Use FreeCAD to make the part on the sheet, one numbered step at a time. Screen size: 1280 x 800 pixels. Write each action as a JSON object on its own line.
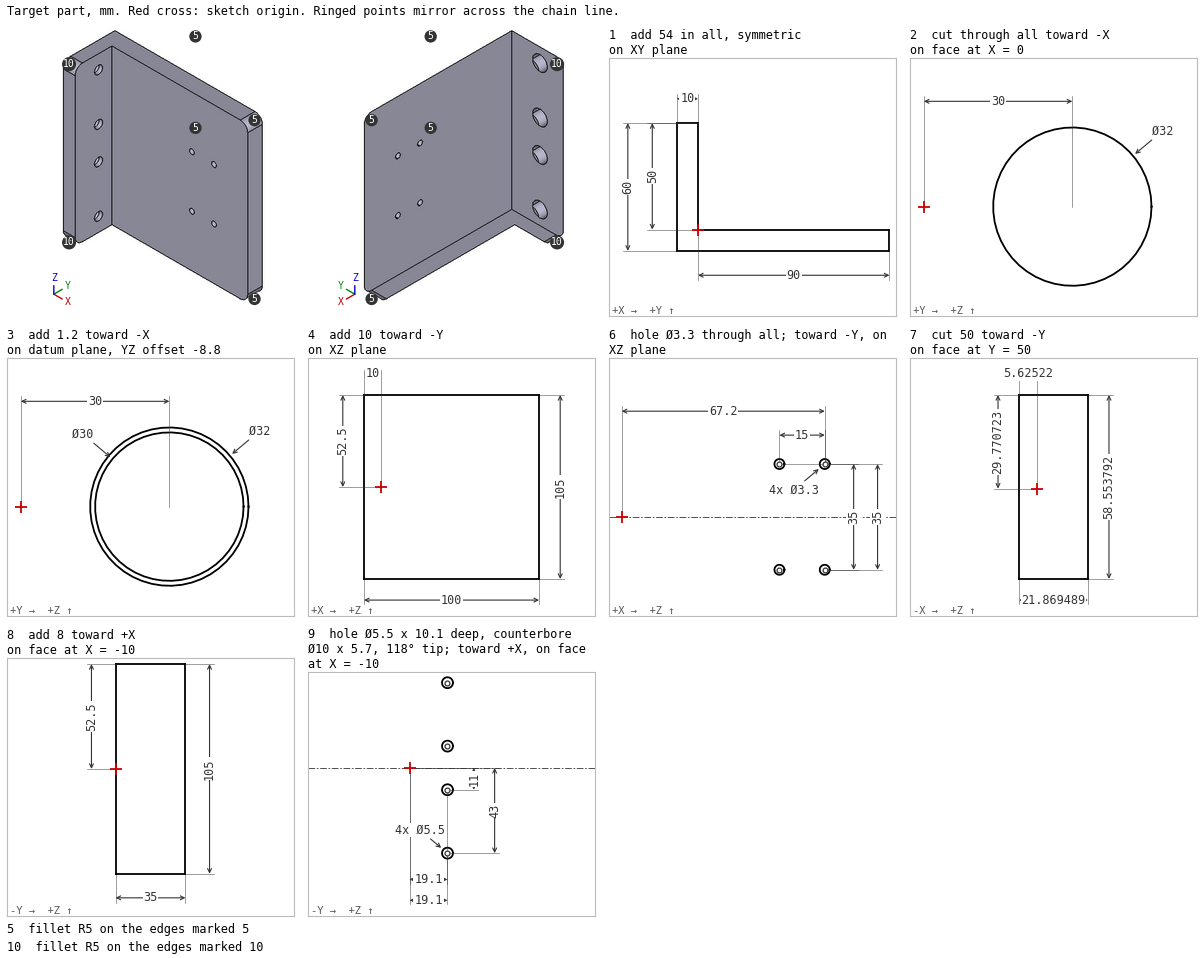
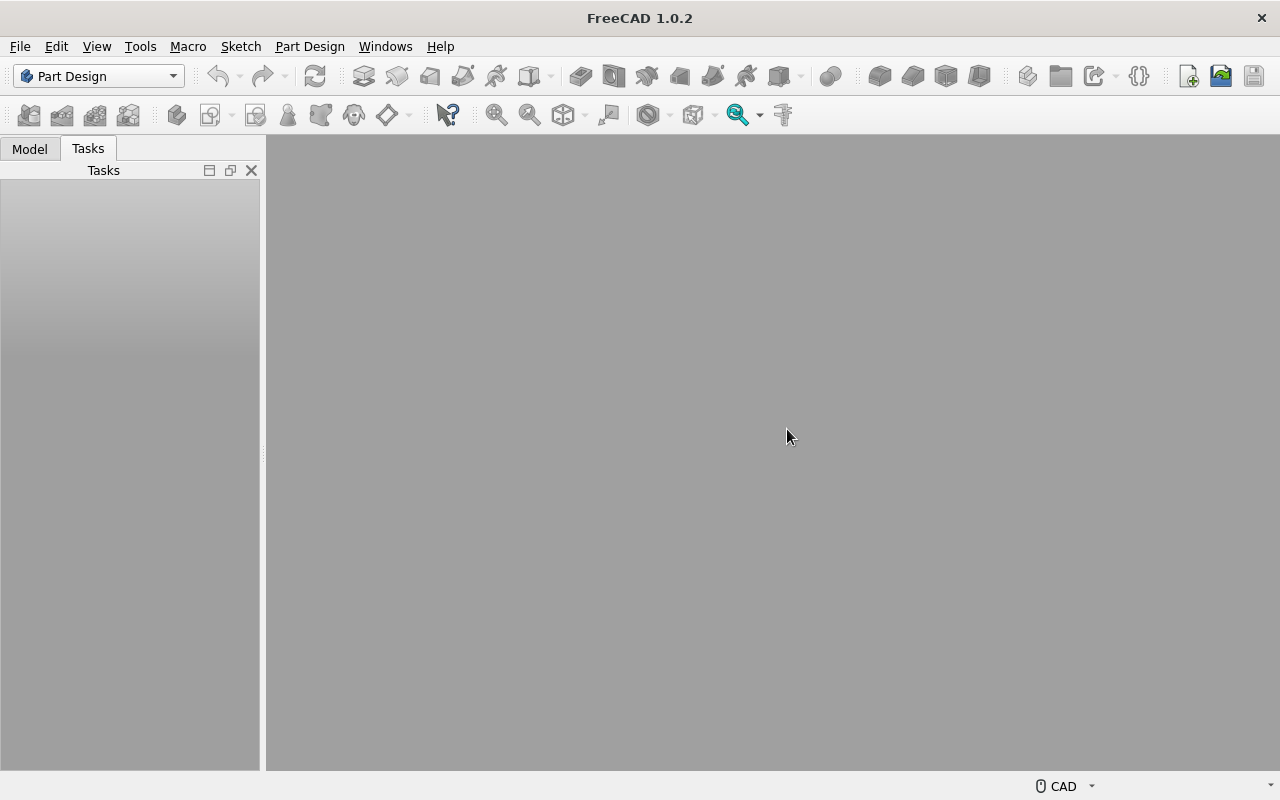
{"action": "left_click", "coordinate": [1188, 76]}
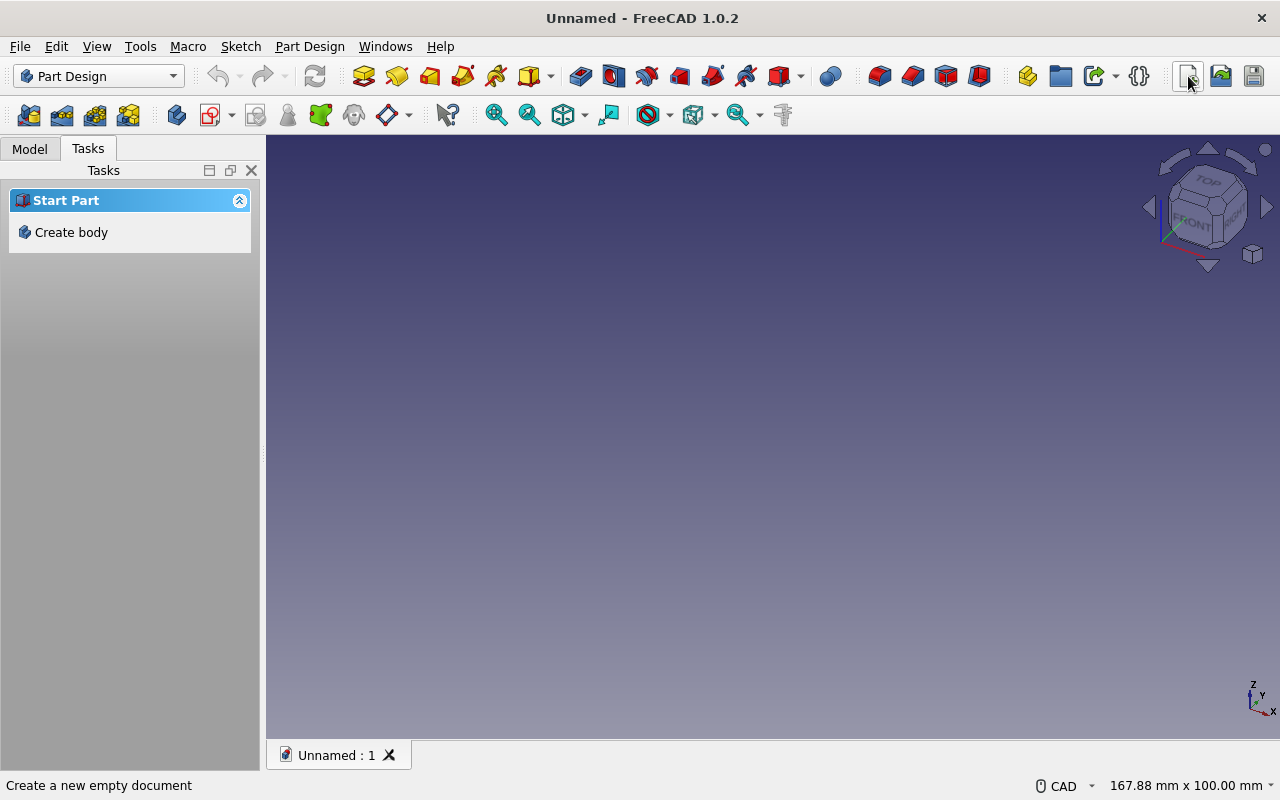
{"action": "left_click", "coordinate": [210, 116]}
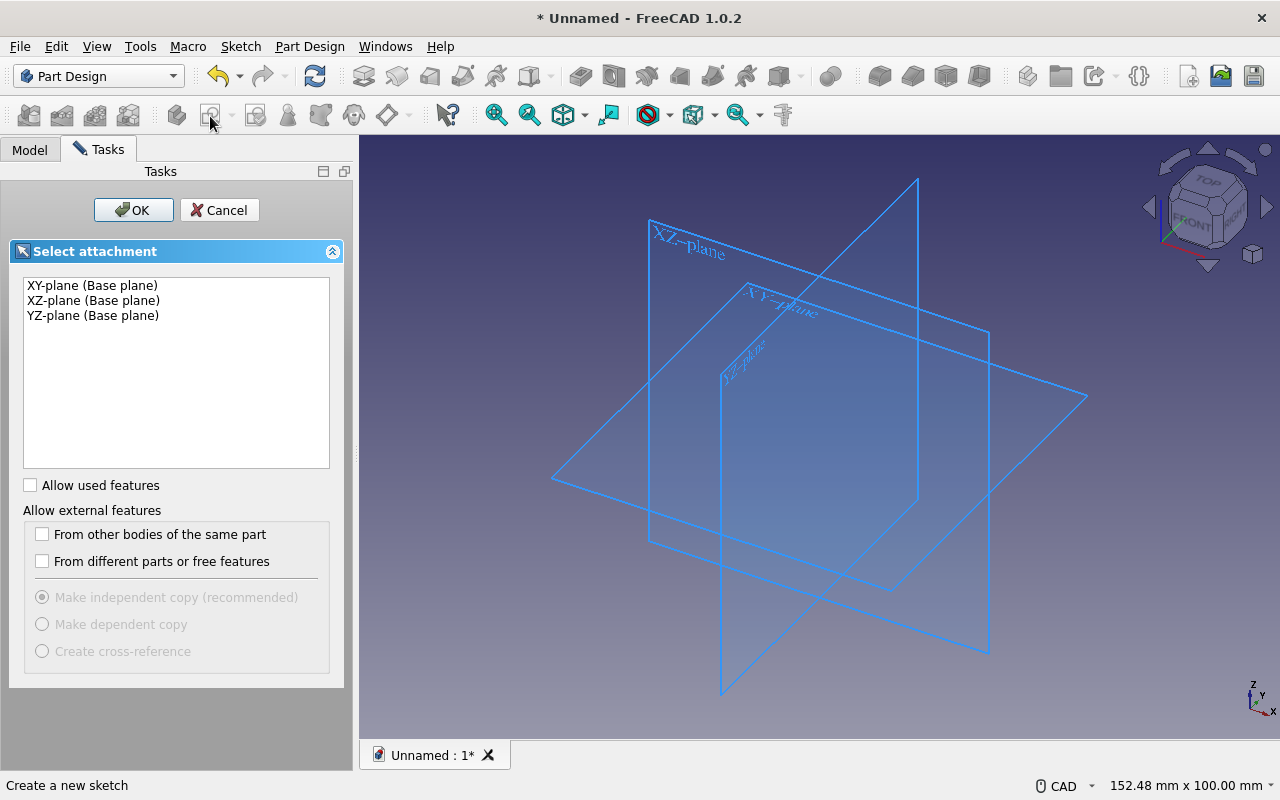
{"action": "left_click", "coordinate": [84, 286]}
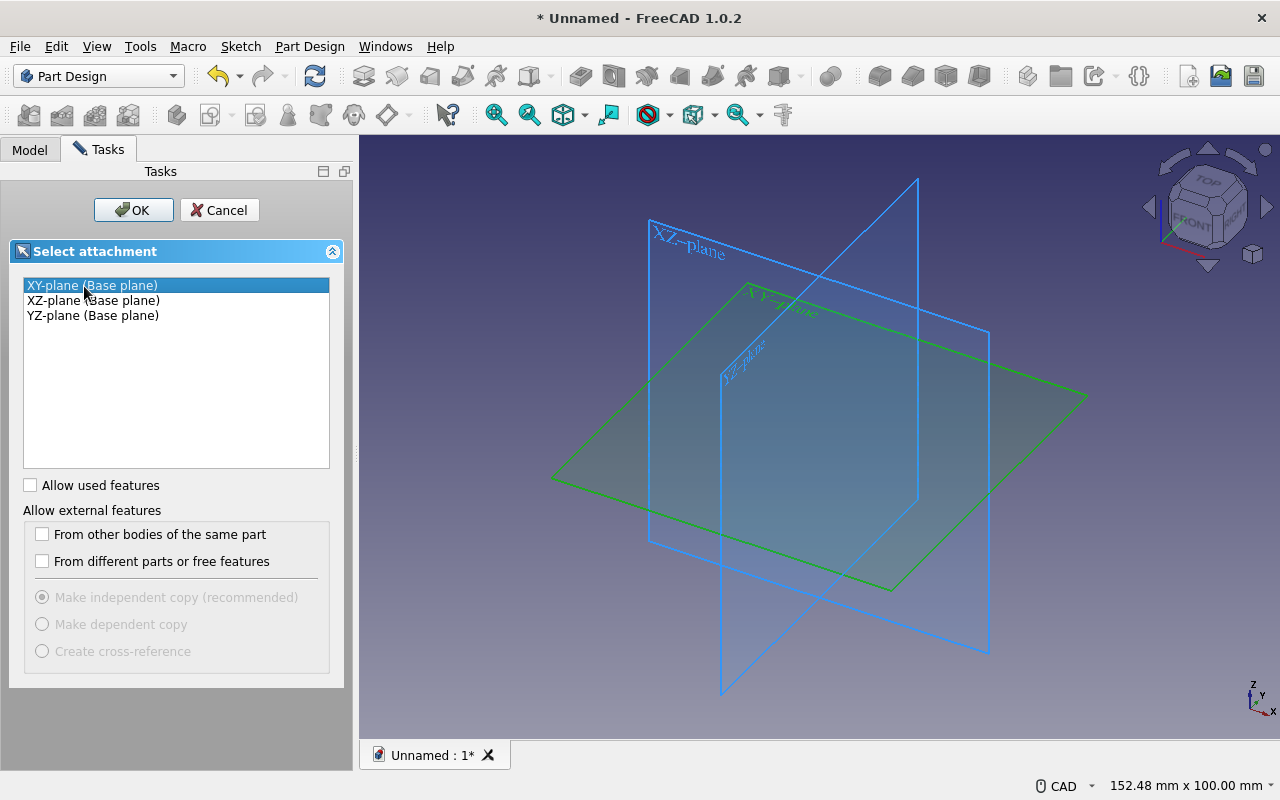
{"action": "left_click", "coordinate": [134, 210]}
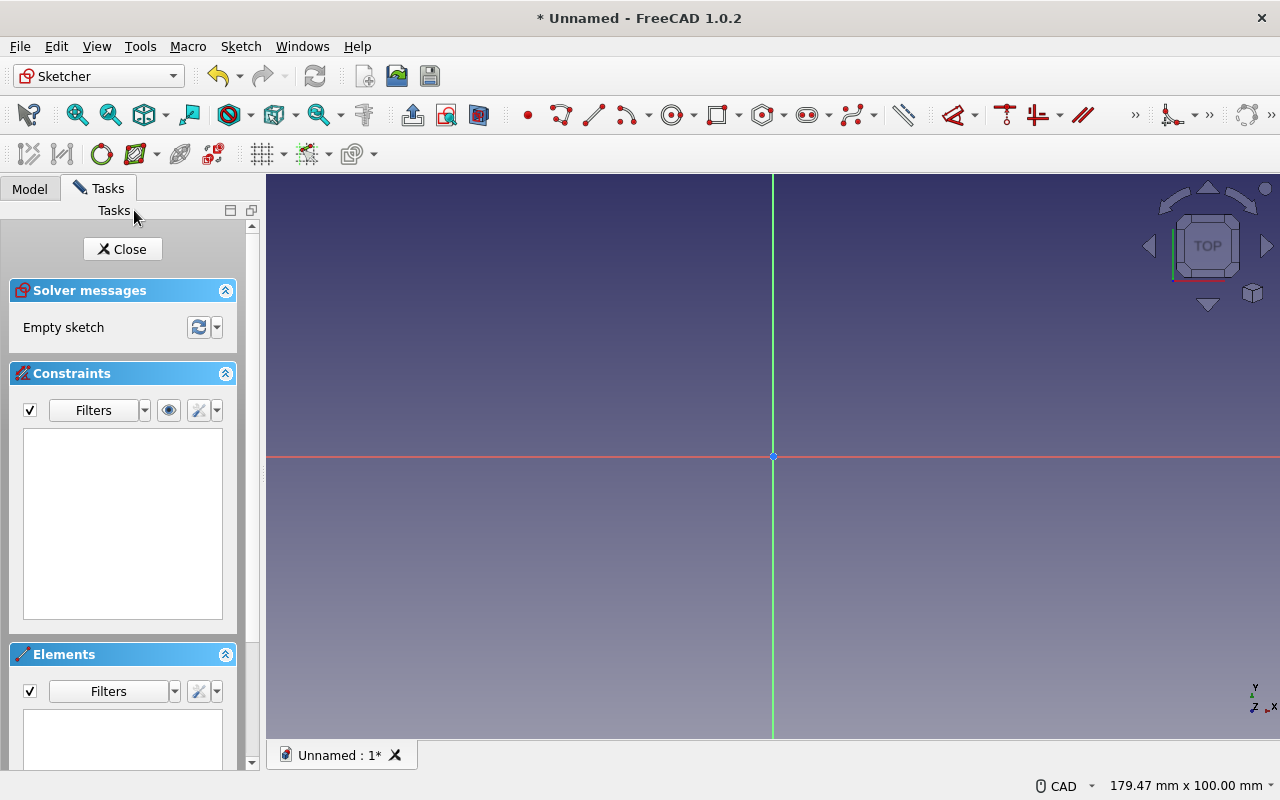
{"action": "scroll", "coordinate": [294, 686], "scroll_direction": "down", "scroll_amount": 2}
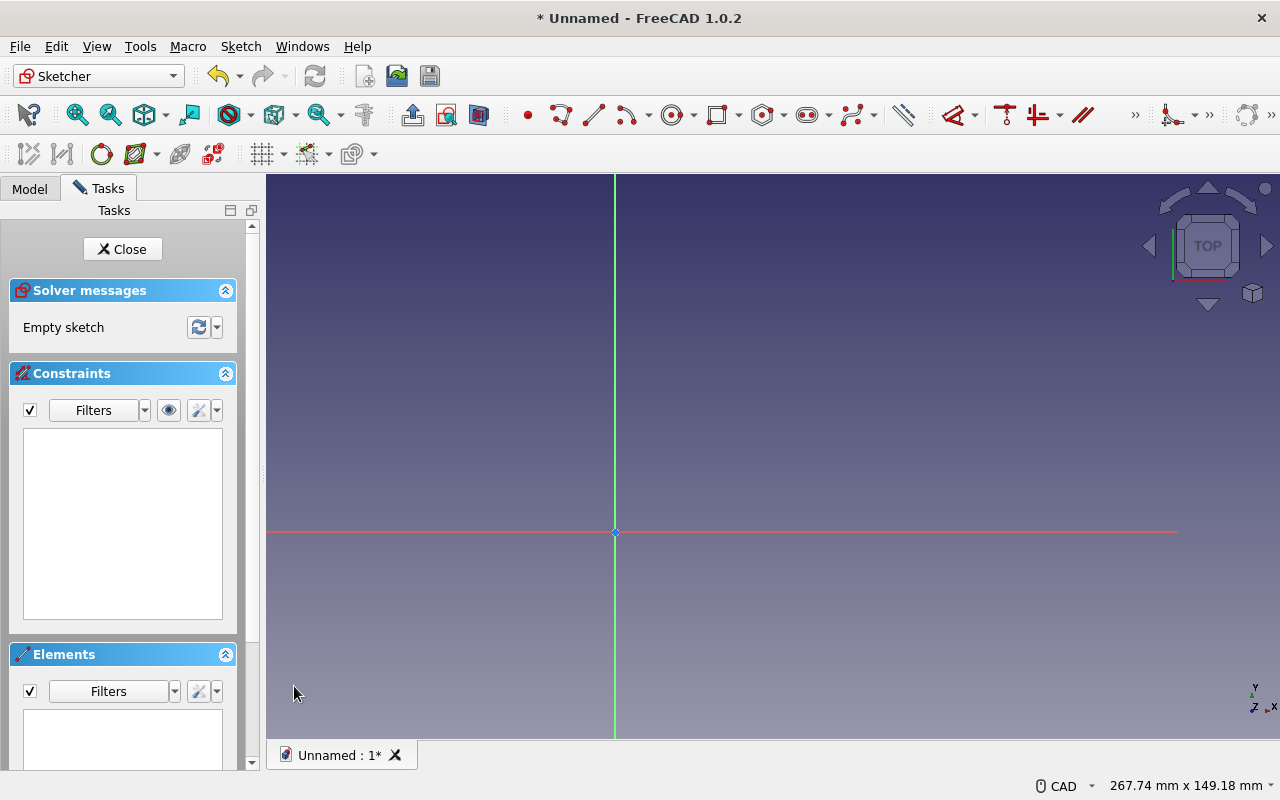
{"action": "scroll", "coordinate": [893, 457], "scroll_direction": "up", "scroll_amount": 2}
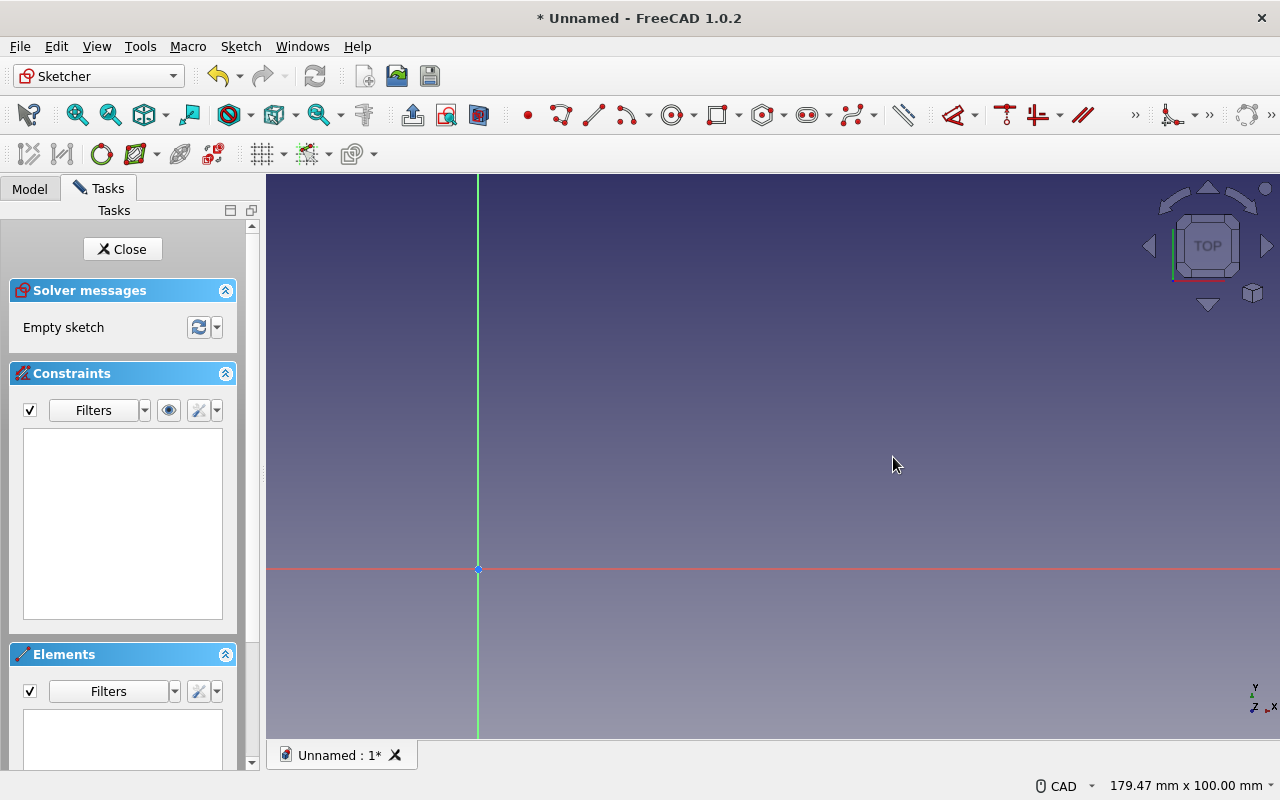
{"action": "left_click", "coordinate": [561, 116]}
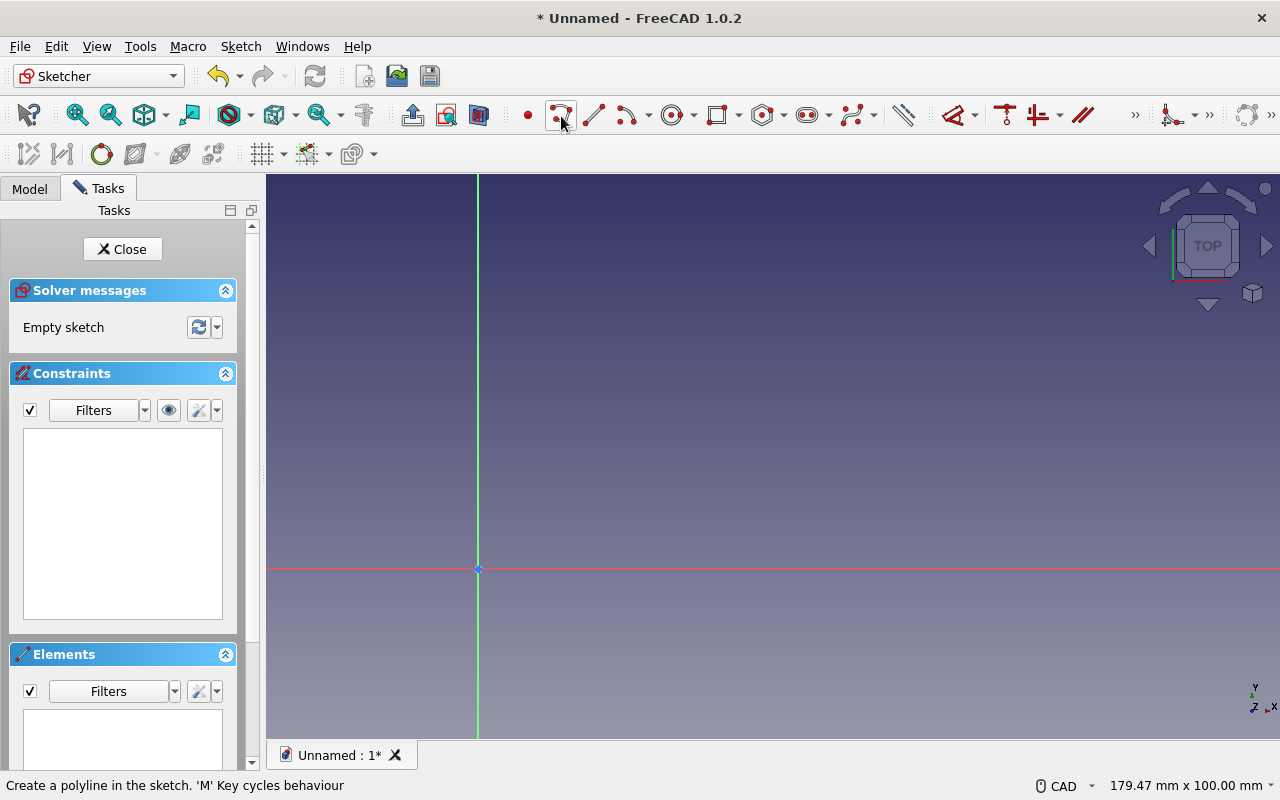
{"action": "left_click", "coordinate": [478, 569]}
{"action": "left_click", "coordinate": [487, 287]}
{"action": "left_click", "coordinate": [422, 287]}
{"action": "left_click", "coordinate": [422, 626]}
{"action": "left_click", "coordinate": [987, 626]}
{"action": "left_click", "coordinate": [987, 560]}
{"action": "left_click", "coordinate": [478, 569]}
{"action": "key", "text": "Escape"}
{"action": "key", "text": "Escape"}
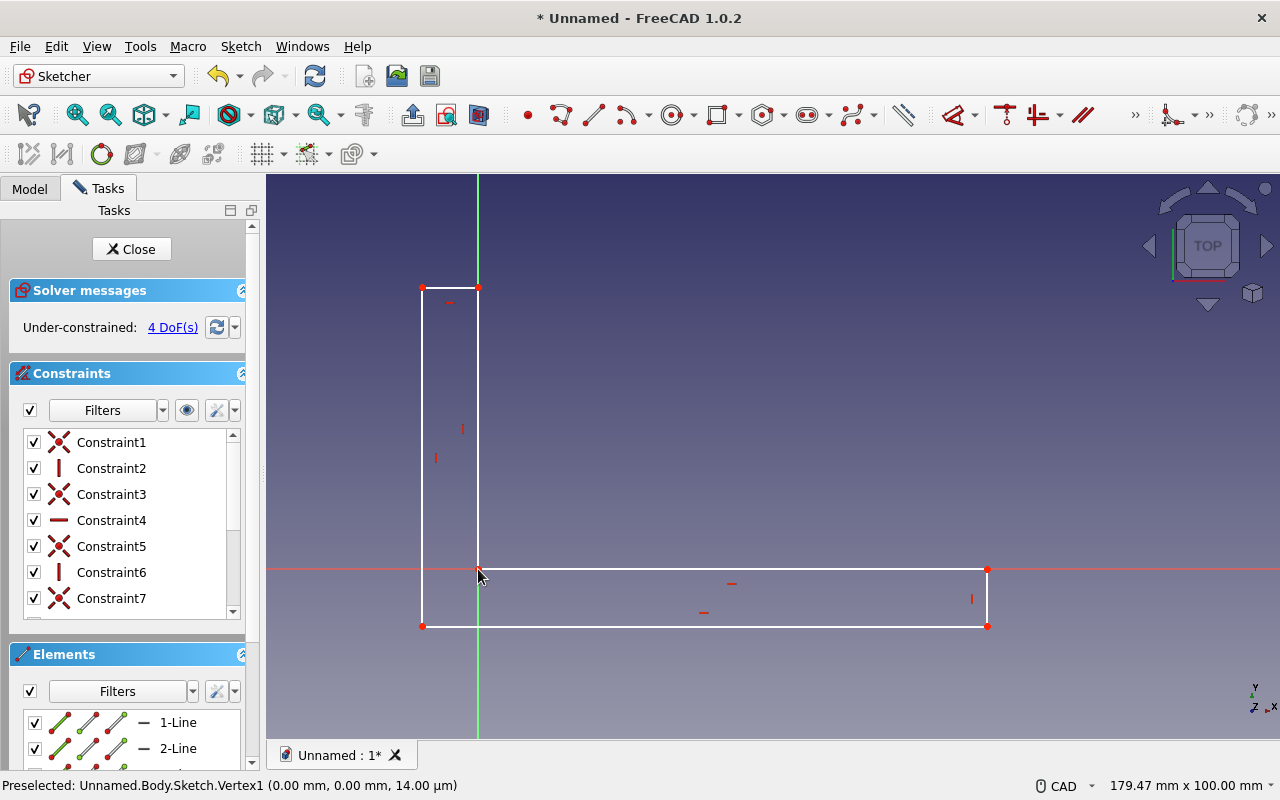
{"action": "left_click", "coordinate": [952, 116]}